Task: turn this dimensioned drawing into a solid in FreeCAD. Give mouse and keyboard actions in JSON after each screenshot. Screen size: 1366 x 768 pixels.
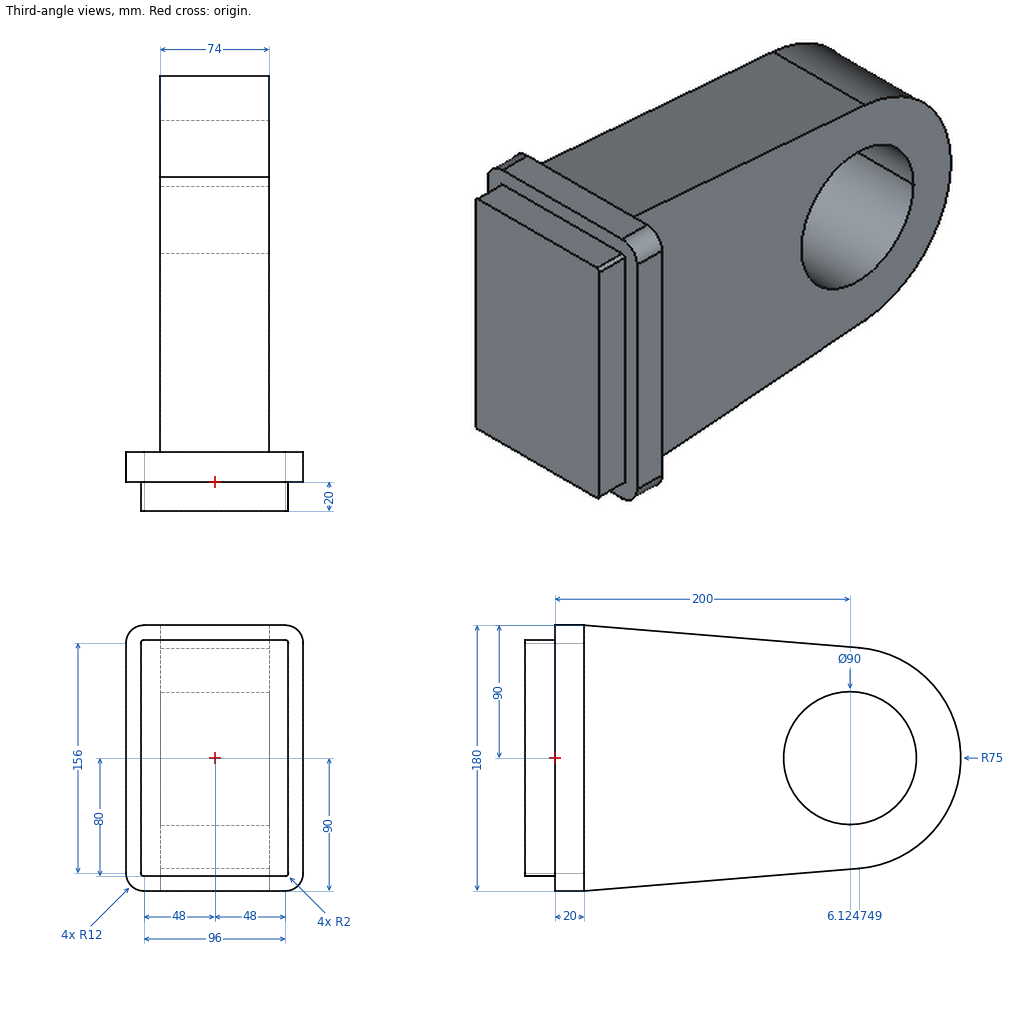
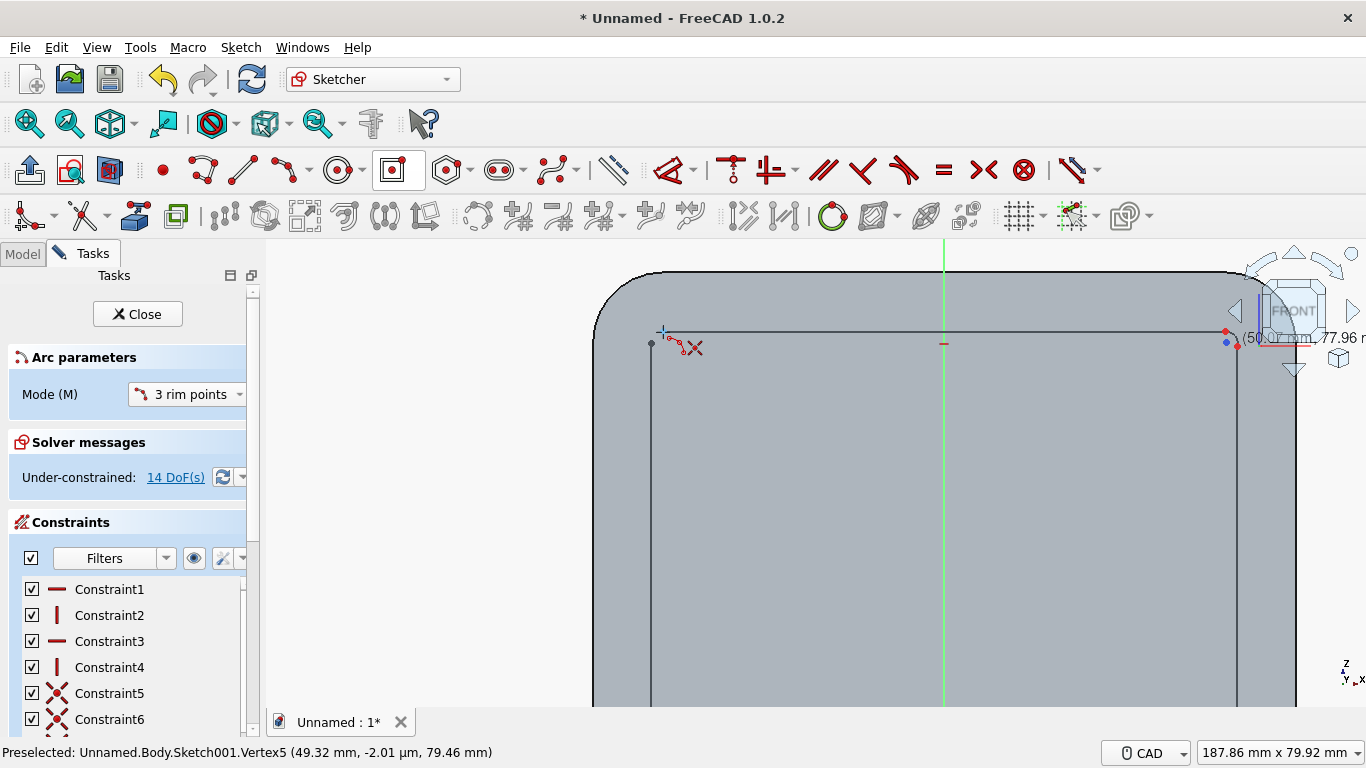
{"action": "left_click", "coordinate": [664, 332]}
{"action": "left_click", "coordinate": [651, 343]}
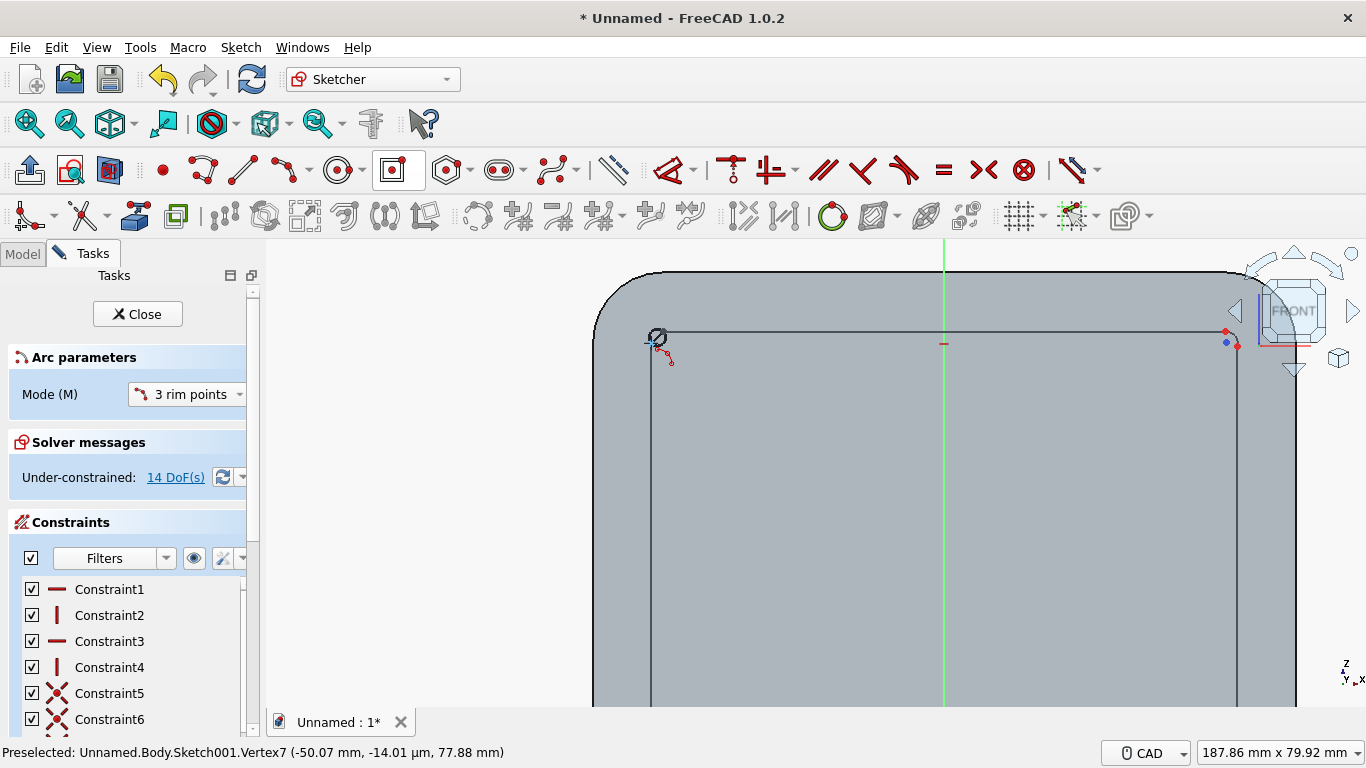
{"action": "scroll", "coordinate": [655, 334], "scroll_direction": "up", "scroll_amount": 8}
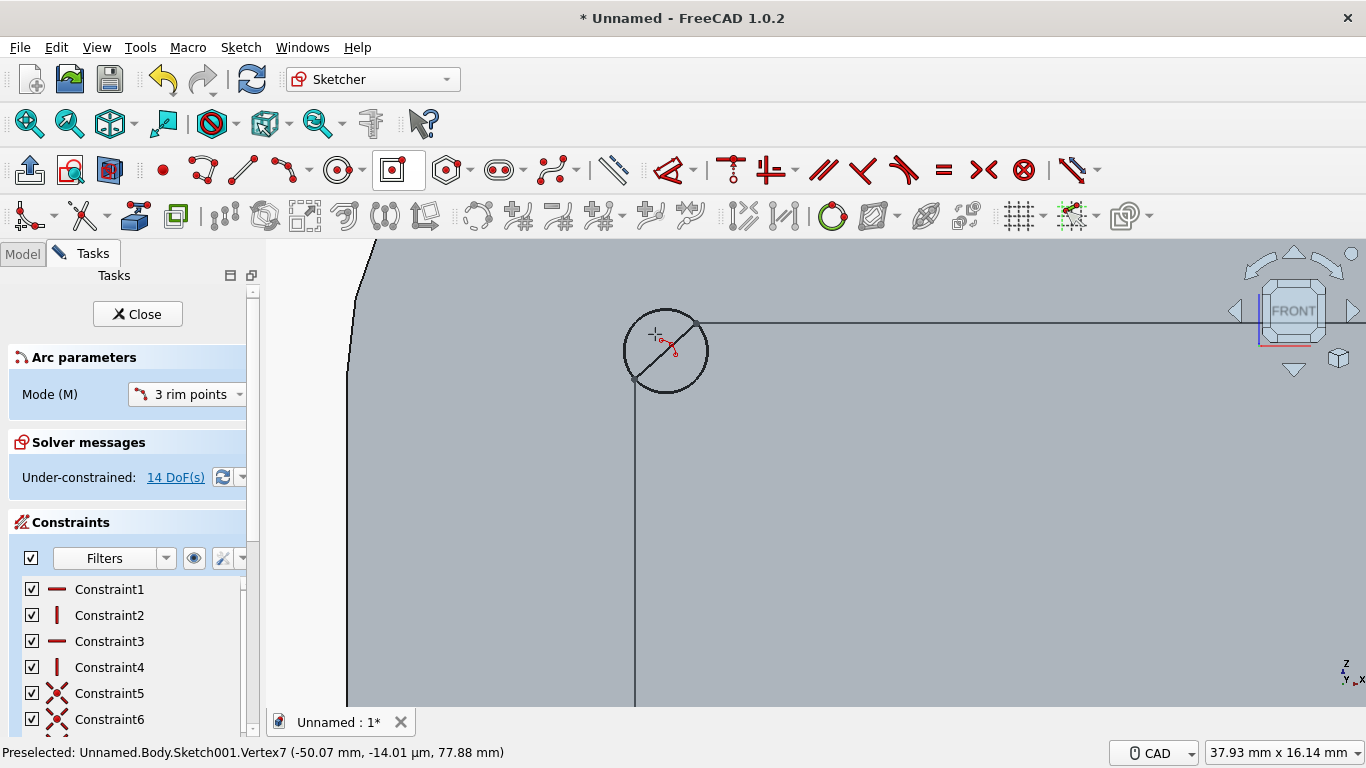
{"action": "left_click", "coordinate": [654, 335]}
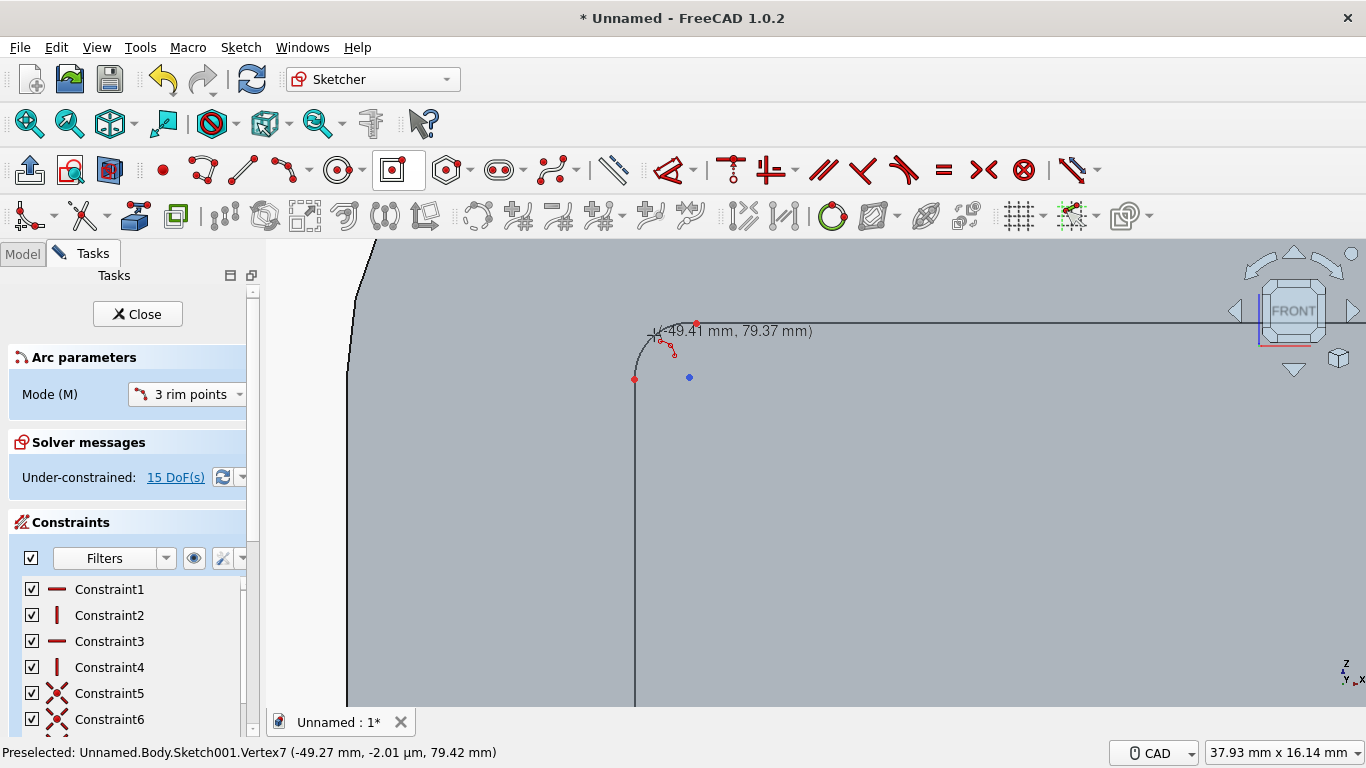
{"action": "scroll", "coordinate": [661, 333], "scroll_direction": "down", "scroll_amount": 14}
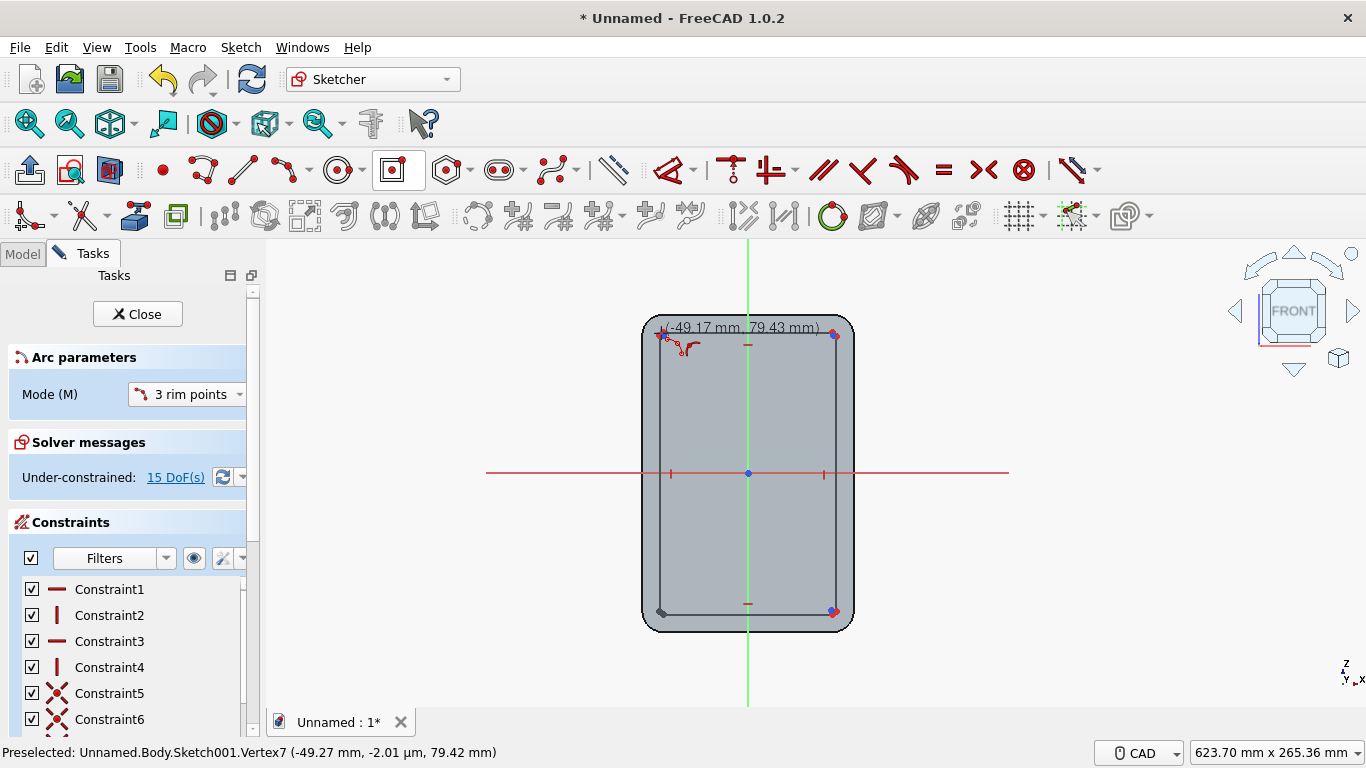
{"action": "scroll", "coordinate": [660, 611], "scroll_direction": "up", "scroll_amount": 6}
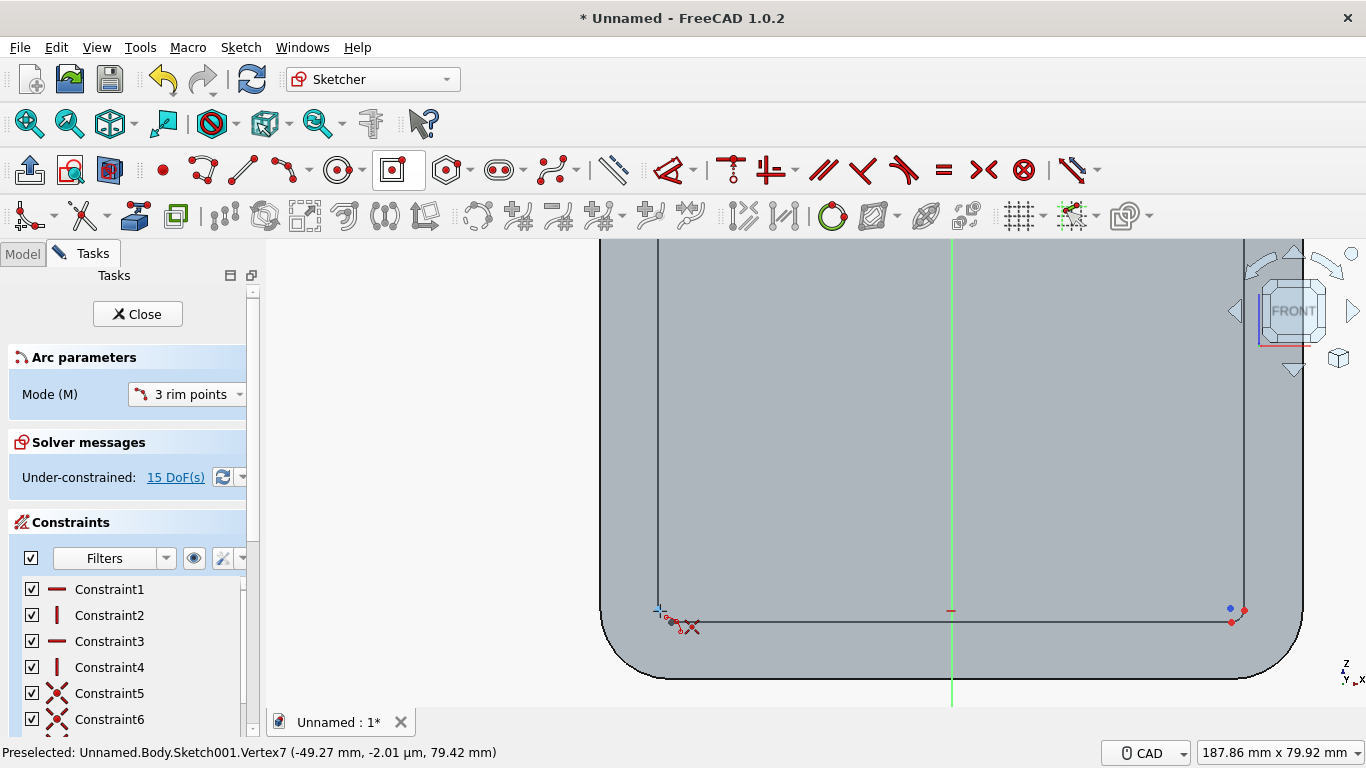
{"action": "left_click", "coordinate": [658, 609]}
{"action": "left_click", "coordinate": [672, 622]}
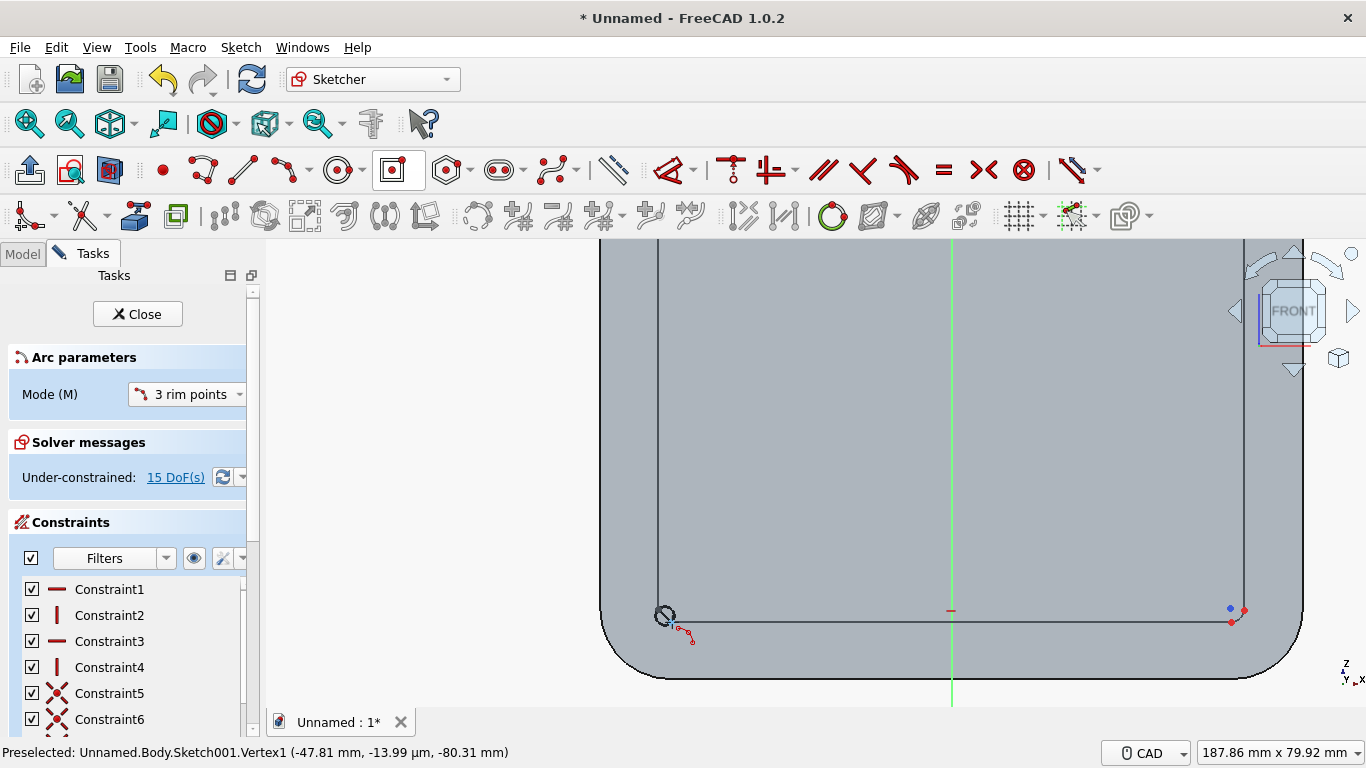
{"action": "scroll", "coordinate": [662, 617], "scroll_direction": "up", "scroll_amount": 8}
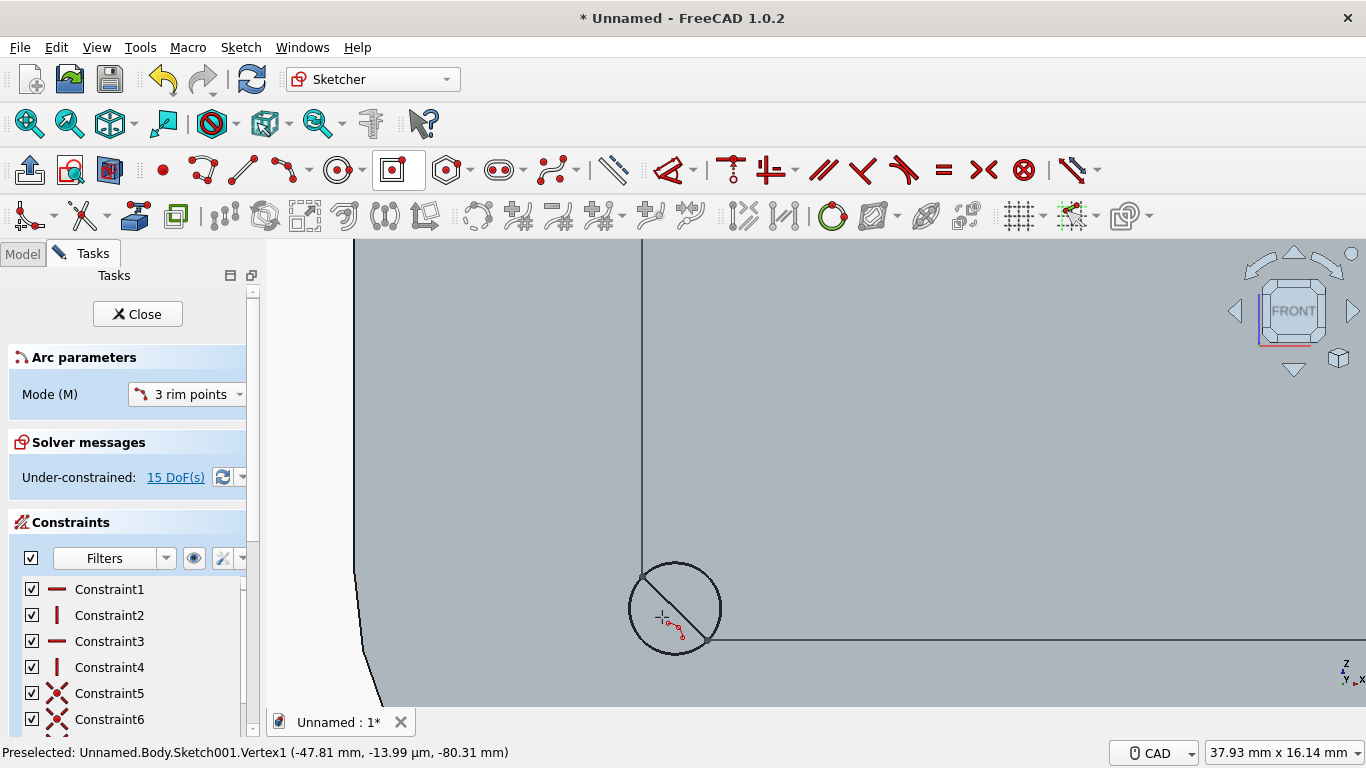
{"action": "left_click", "coordinate": [662, 614]}
{"action": "key", "text": "Escape"}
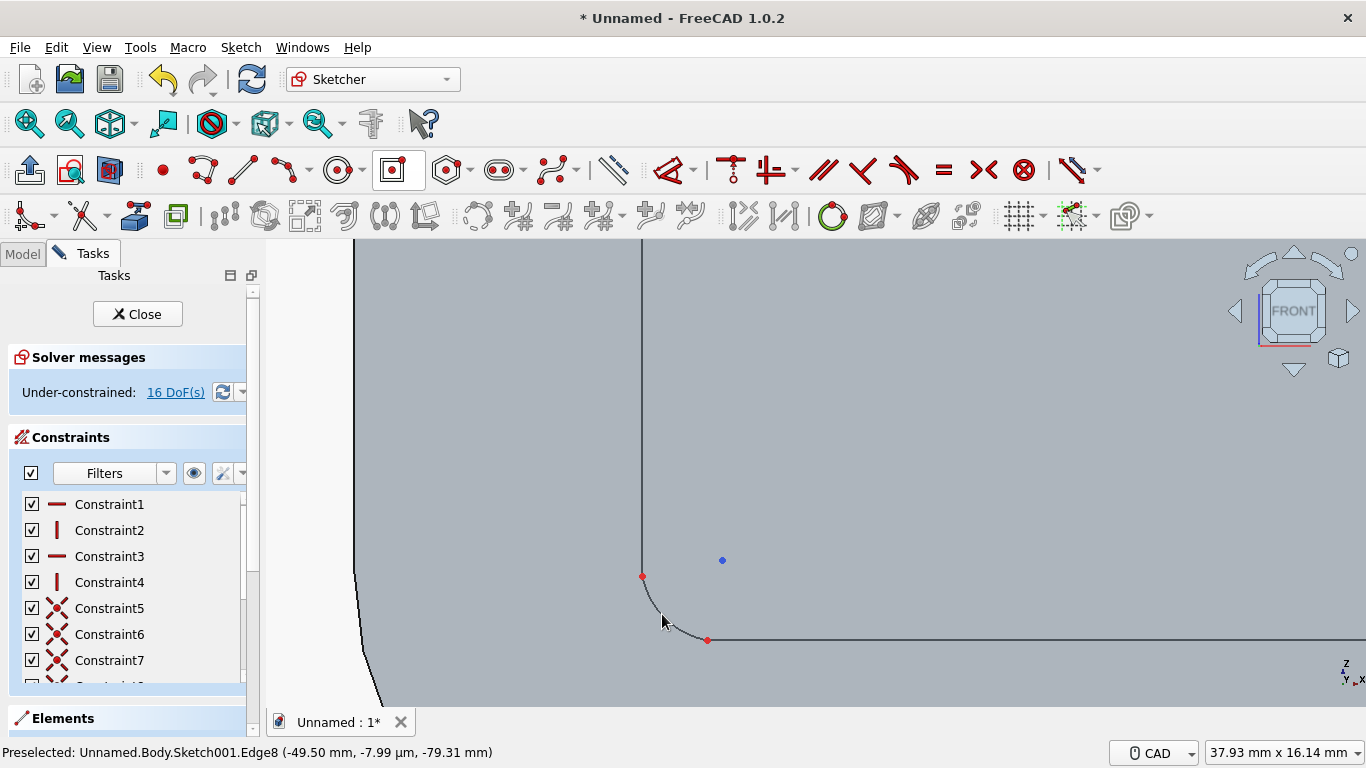
{"action": "scroll", "coordinate": [660, 613], "scroll_direction": "down", "scroll_amount": 14}